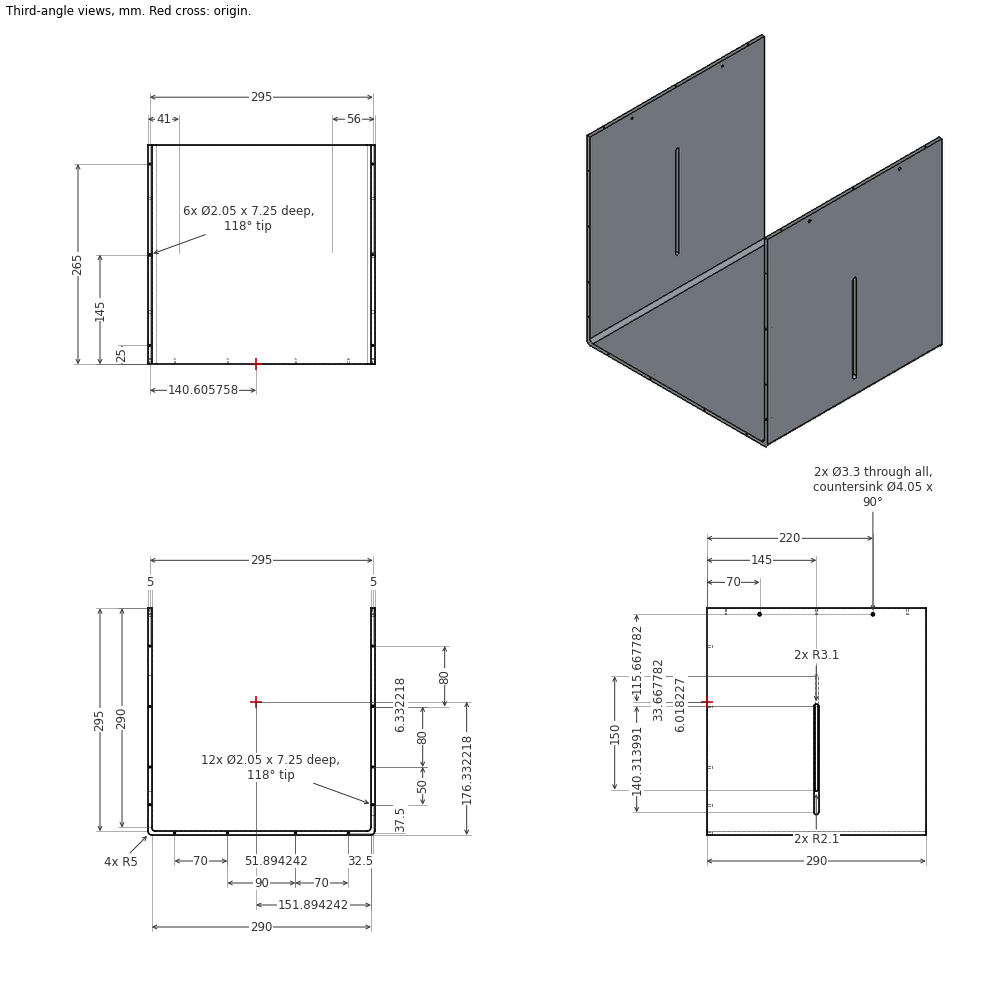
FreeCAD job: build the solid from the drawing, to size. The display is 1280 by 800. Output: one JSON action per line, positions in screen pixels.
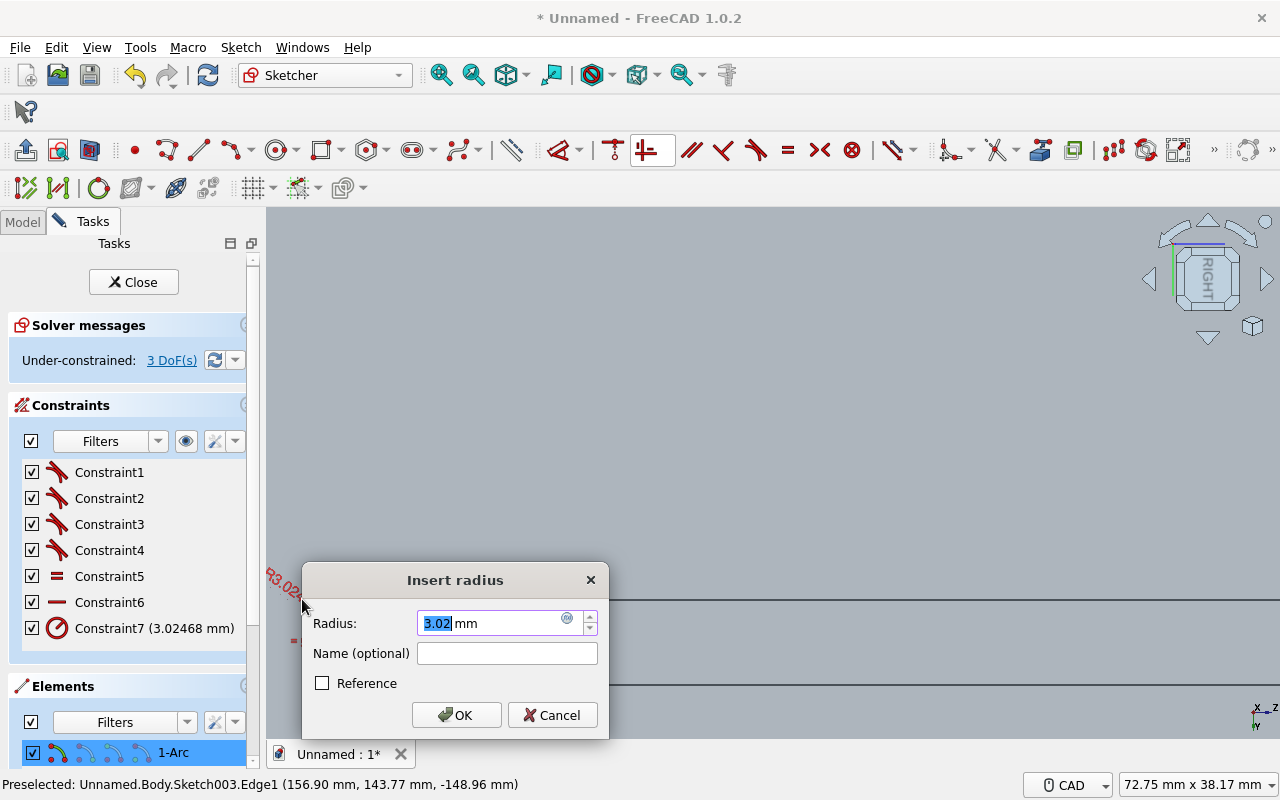
{"action": "type", "text": "3.1"}
{"action": "key", "text": "Return"}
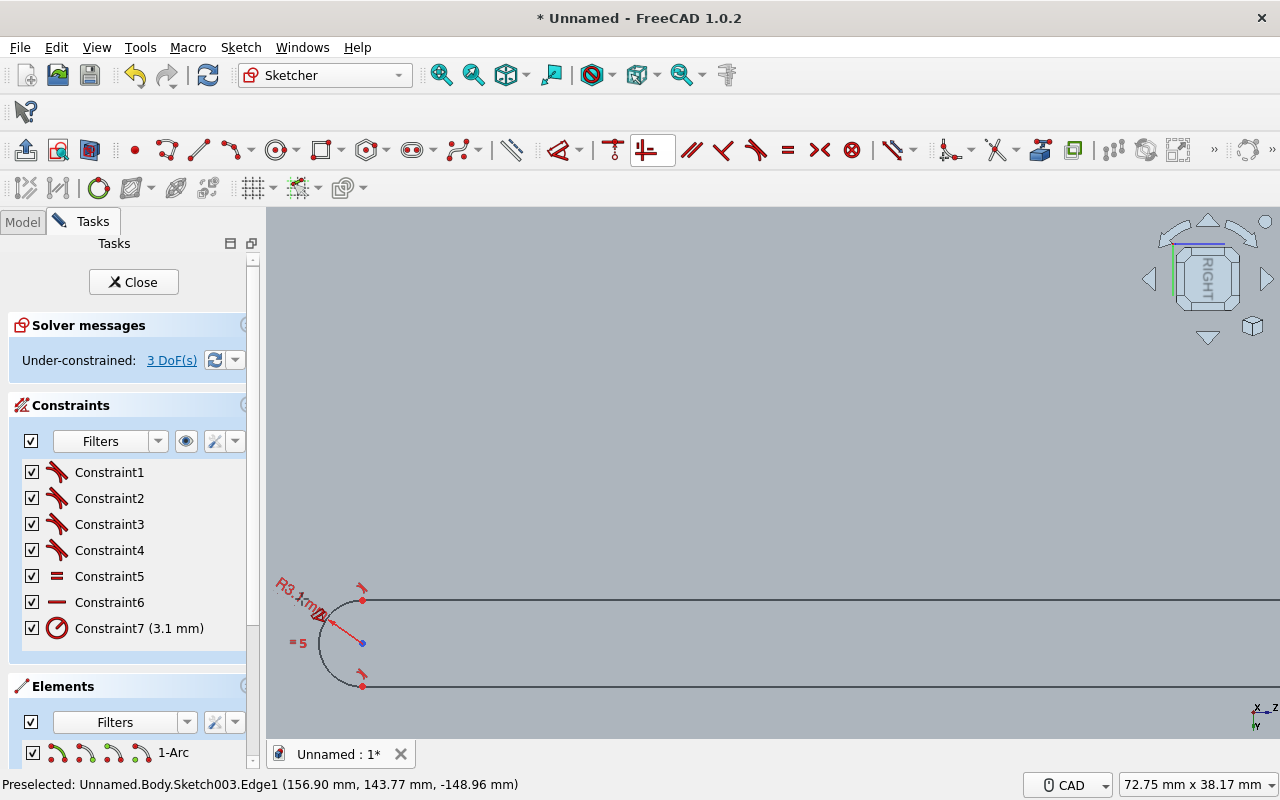
{"action": "scroll", "coordinate": [575, 636], "scroll_direction": "down", "scroll_amount": 9}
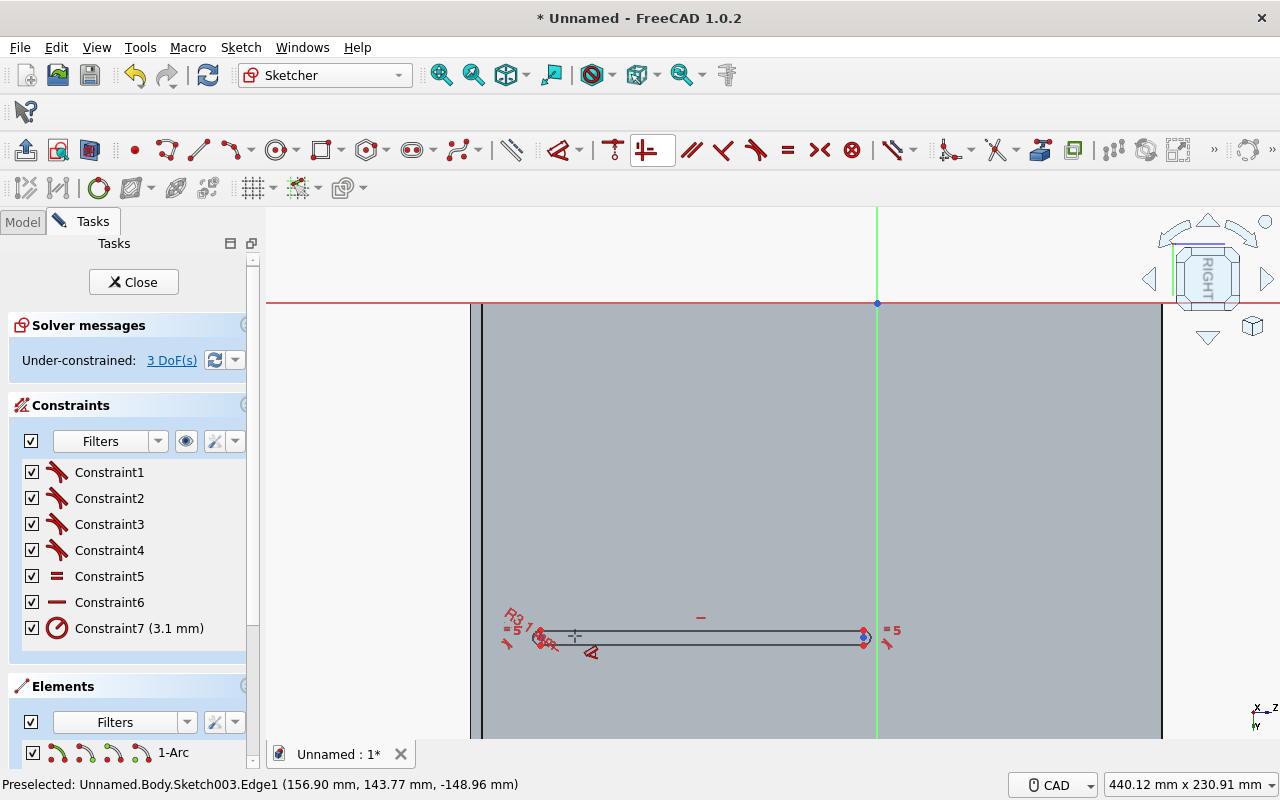
{"action": "scroll", "coordinate": [540, 638], "scroll_direction": "up", "scroll_amount": 3}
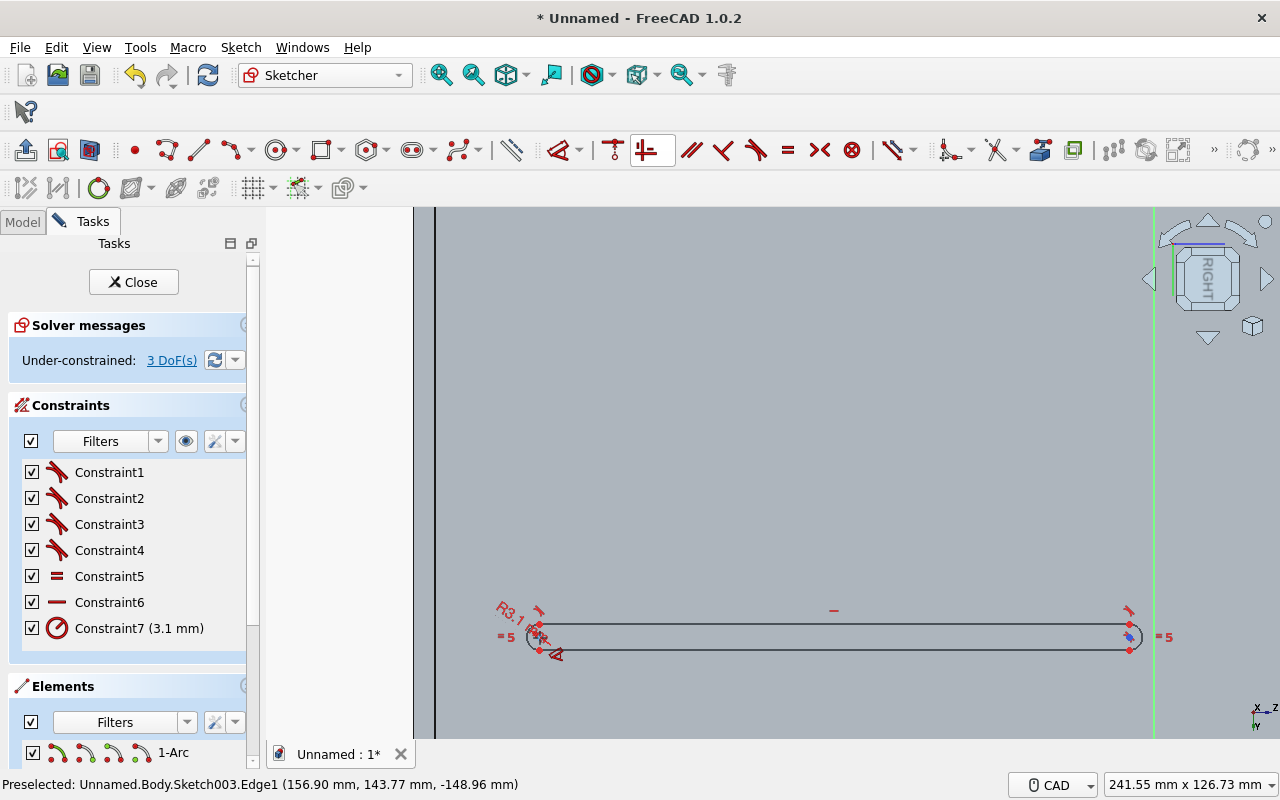
{"action": "left_click", "coordinate": [540, 637]}
{"action": "left_click", "coordinate": [506, 436]}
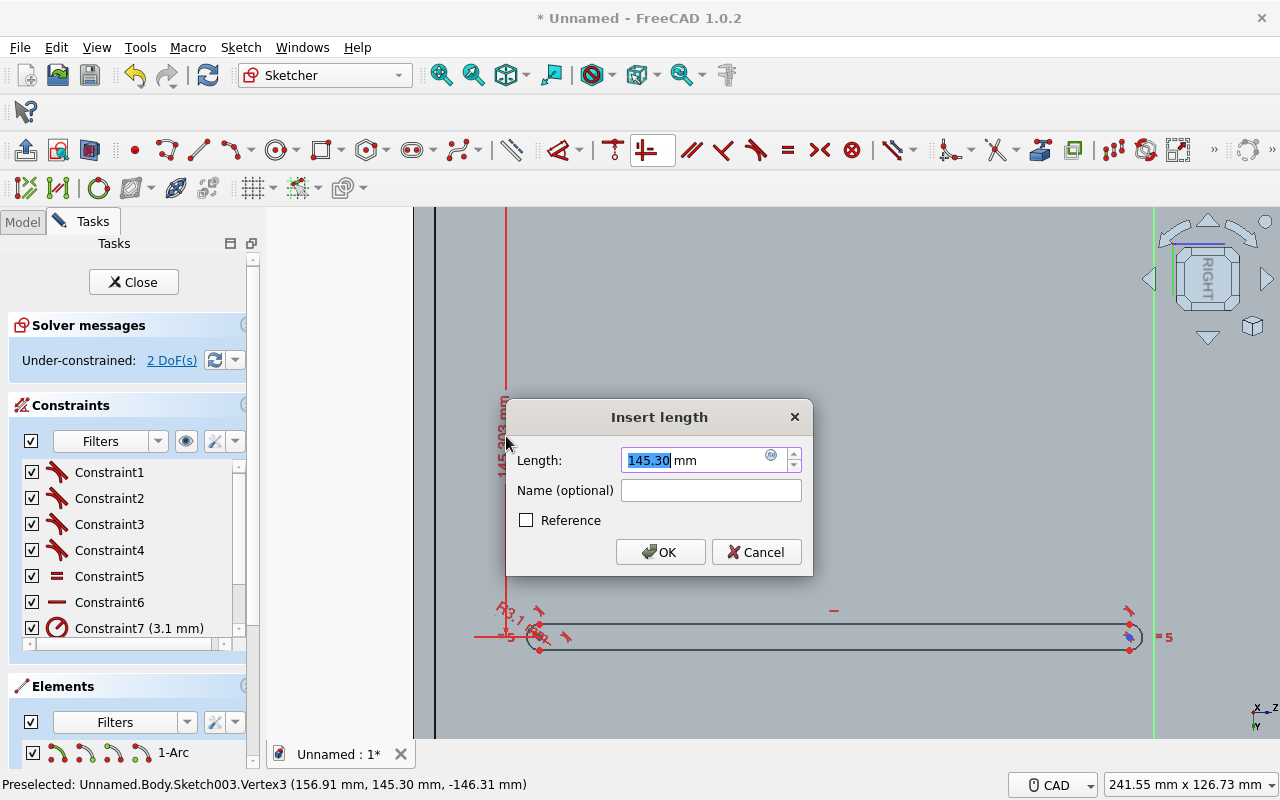
{"action": "type", "text": "145"}
{"action": "key", "text": "Return"}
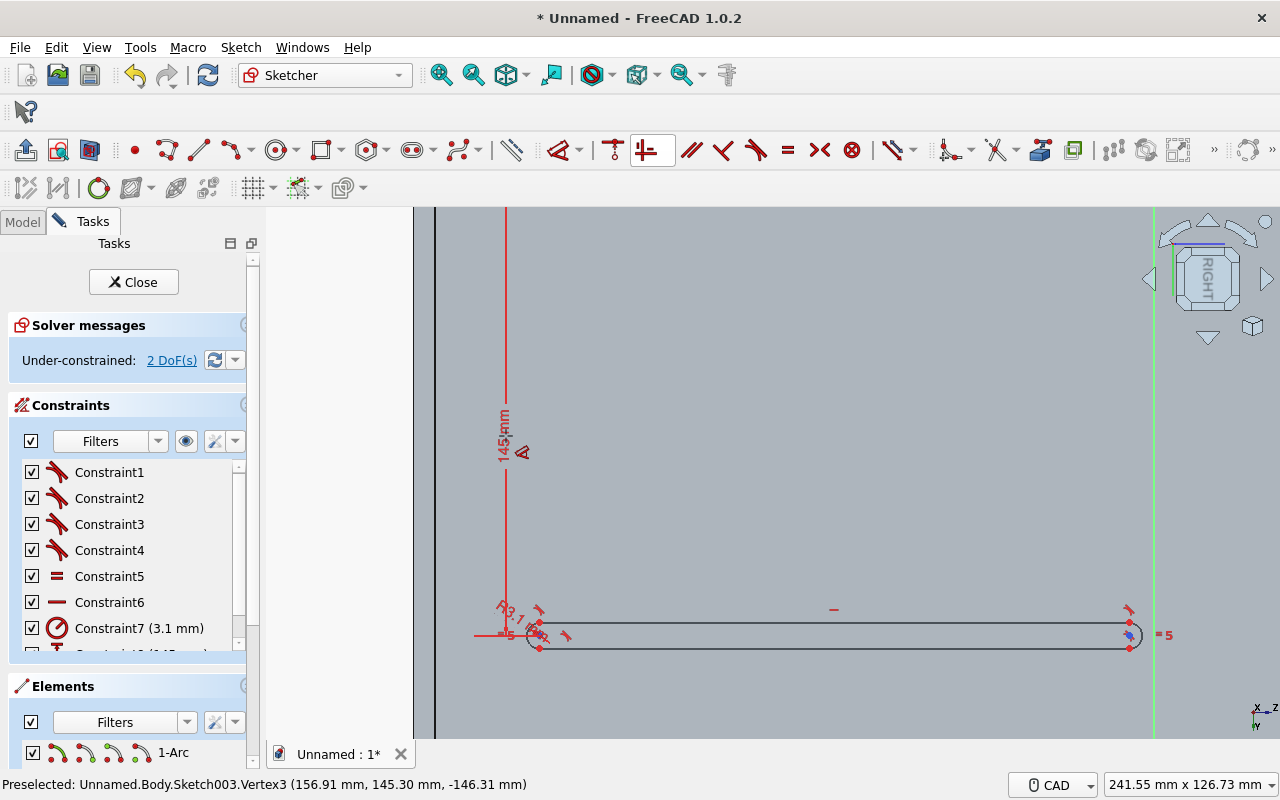
{"action": "scroll", "coordinate": [539, 637], "scroll_direction": "down", "scroll_amount": 3}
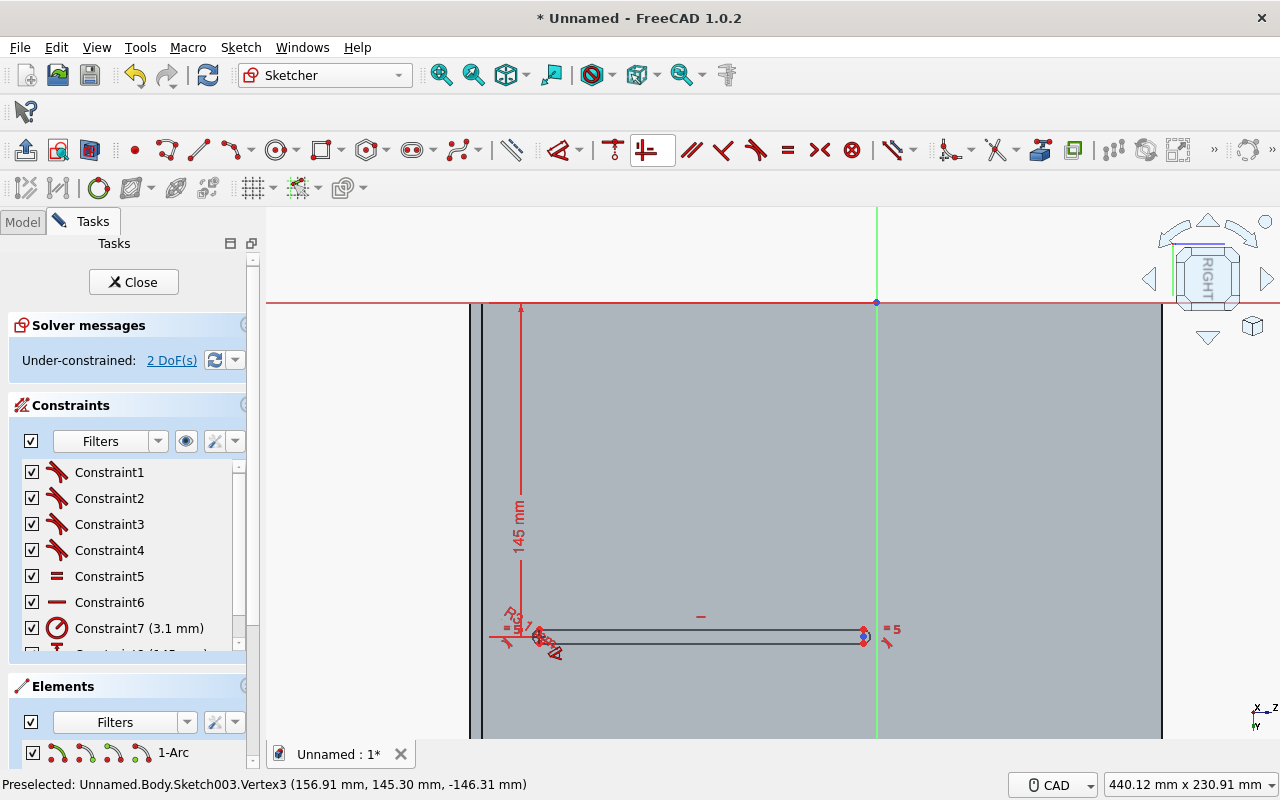
{"action": "scroll", "coordinate": [863, 644], "scroll_direction": "up", "scroll_amount": 6}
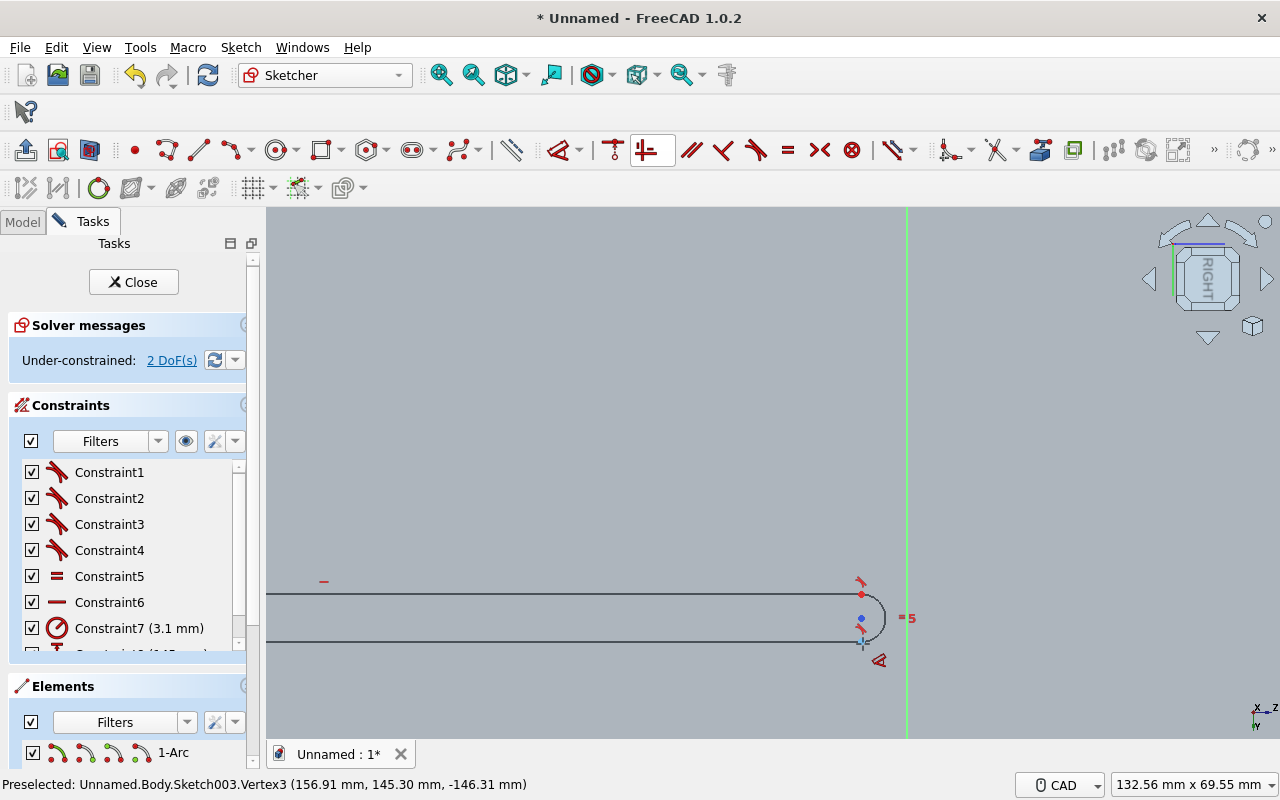
{"action": "left_click", "coordinate": [862, 642]}
{"action": "left_click", "coordinate": [884, 676]}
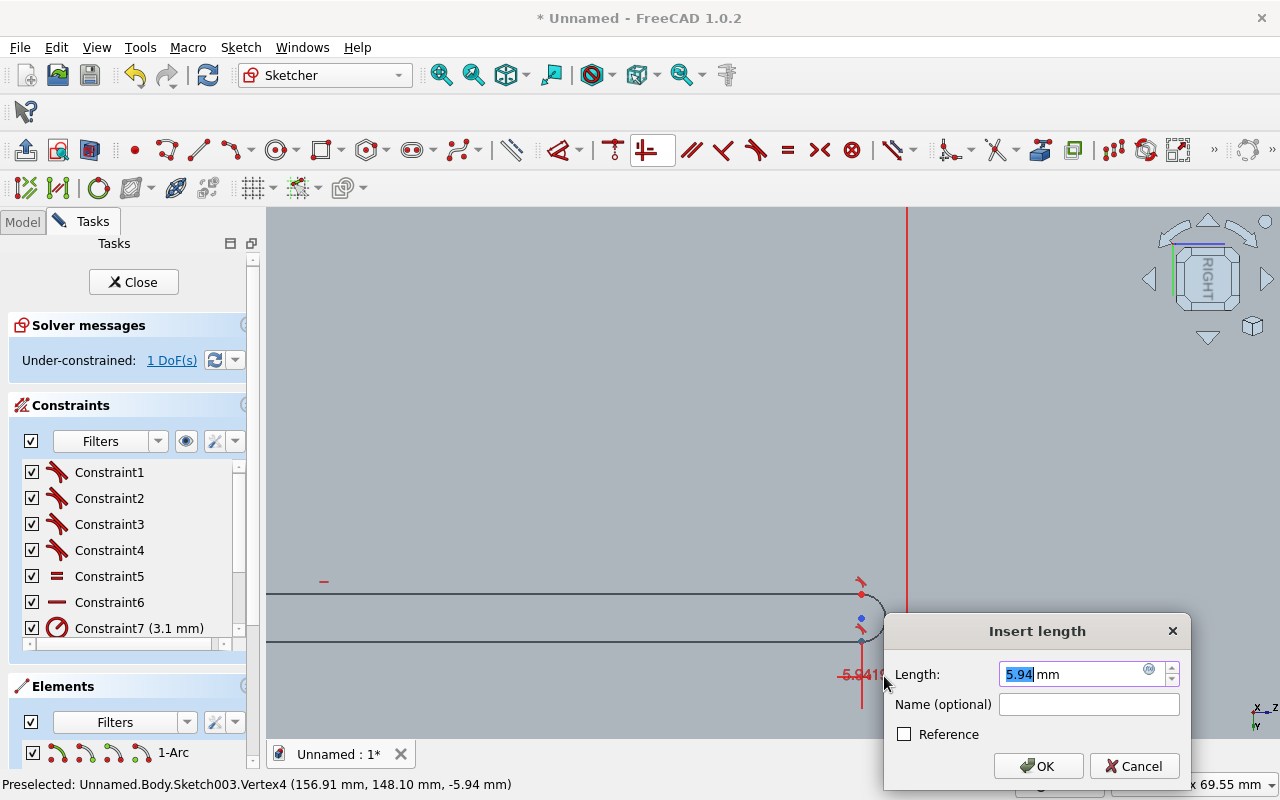
{"action": "type", "text": "6.018227"}
{"action": "key", "text": "Return"}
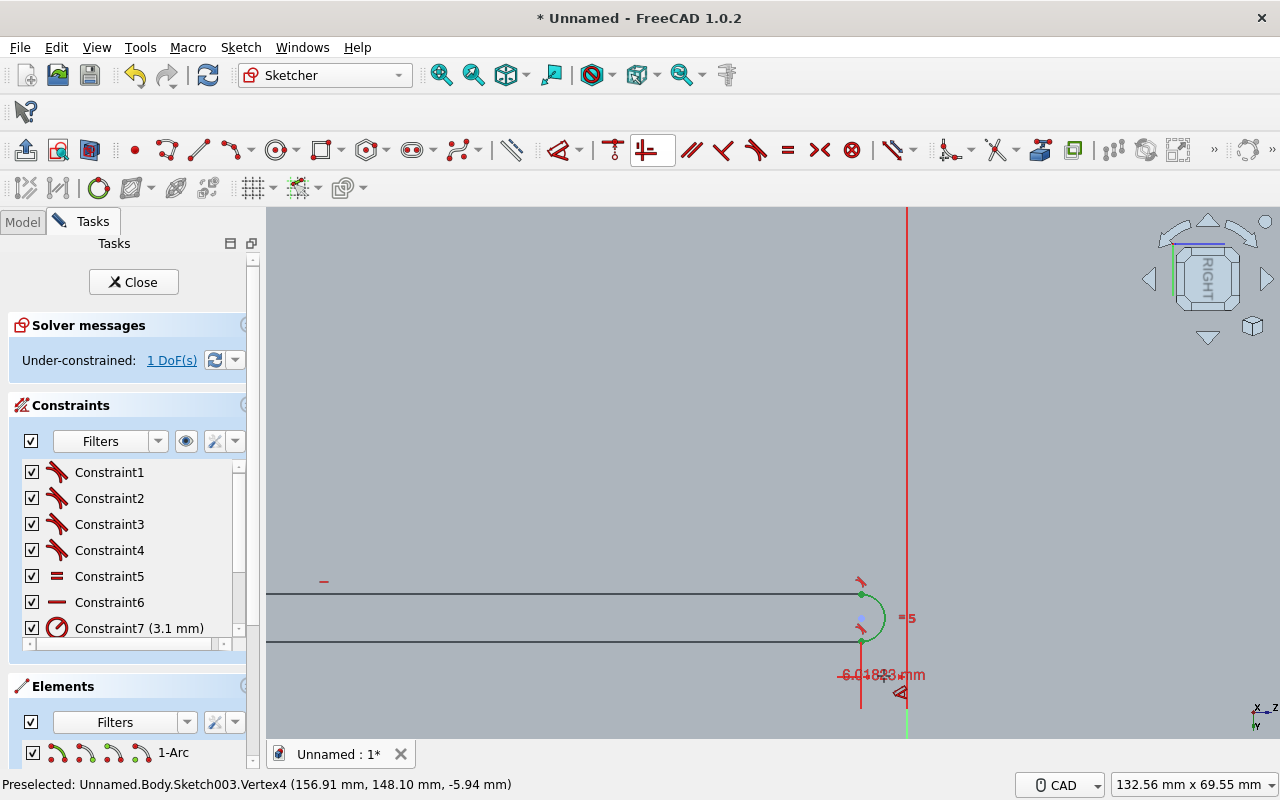
{"action": "left_click", "coordinate": [539, 594]}
{"action": "left_click", "coordinate": [578, 628]}